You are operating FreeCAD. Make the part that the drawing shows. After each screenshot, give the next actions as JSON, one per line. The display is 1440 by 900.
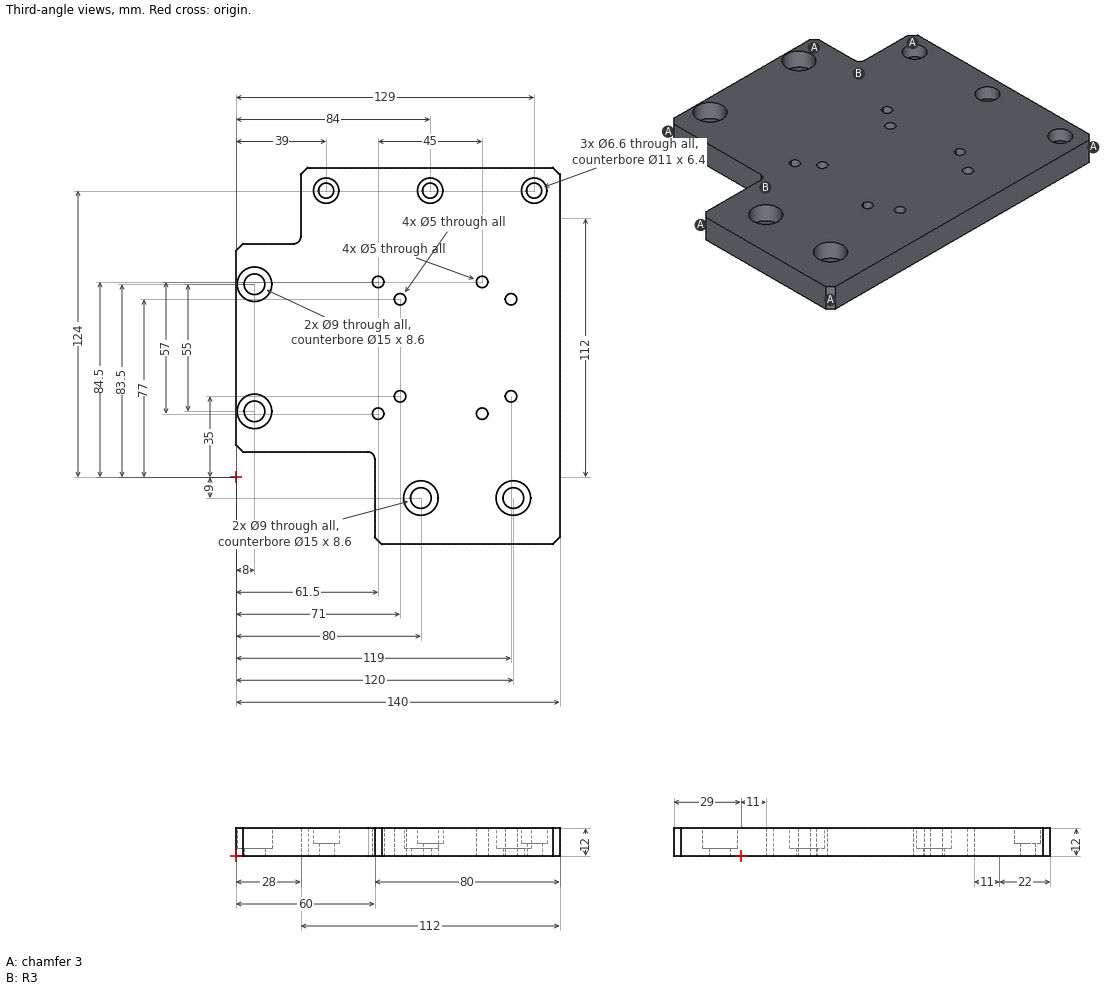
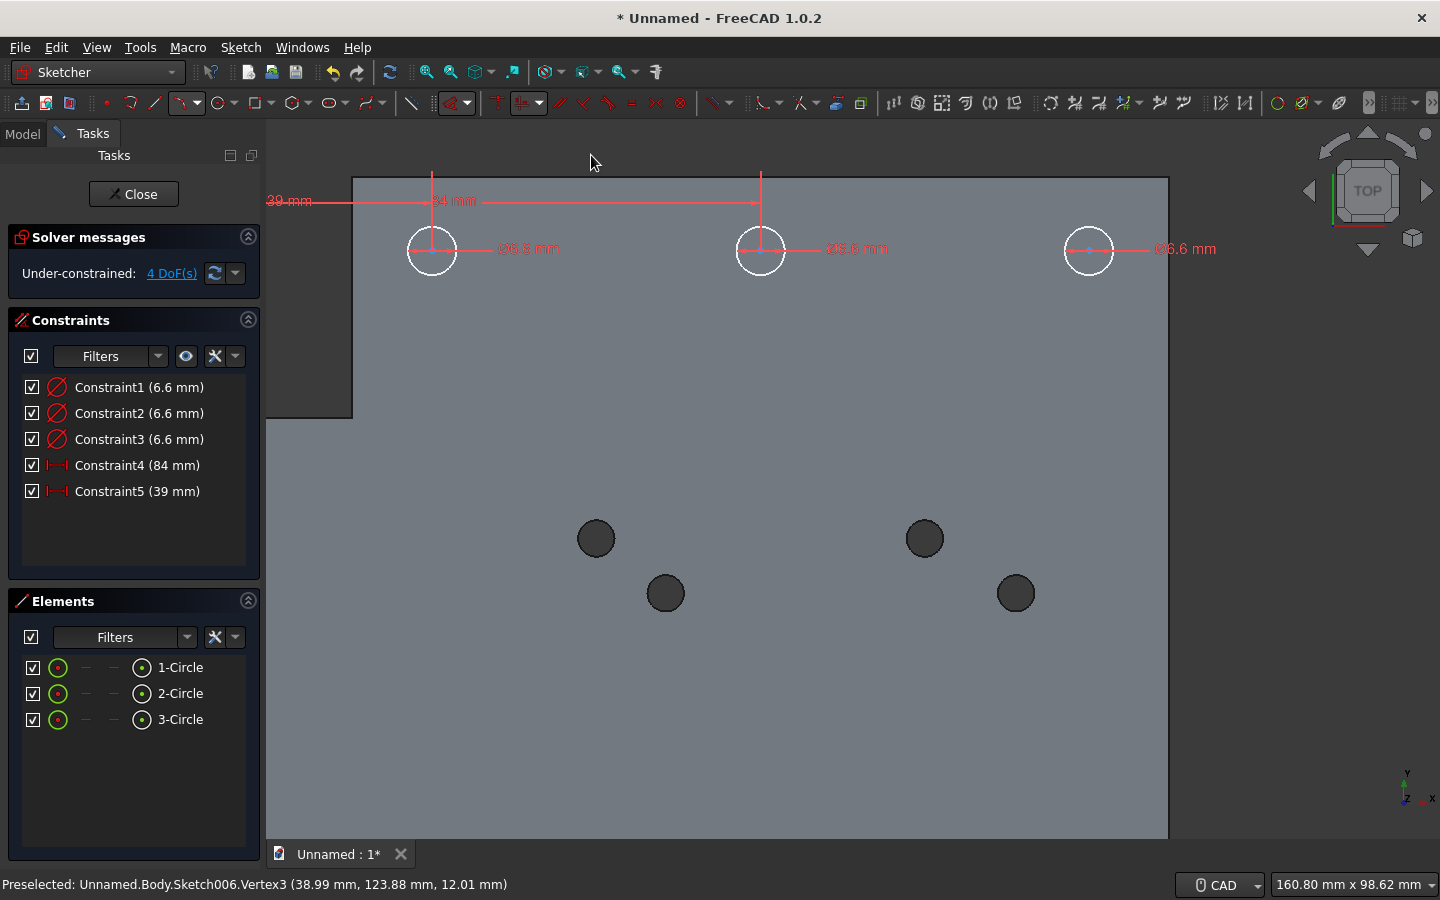
{"action": "left_click", "coordinate": [1089, 251]}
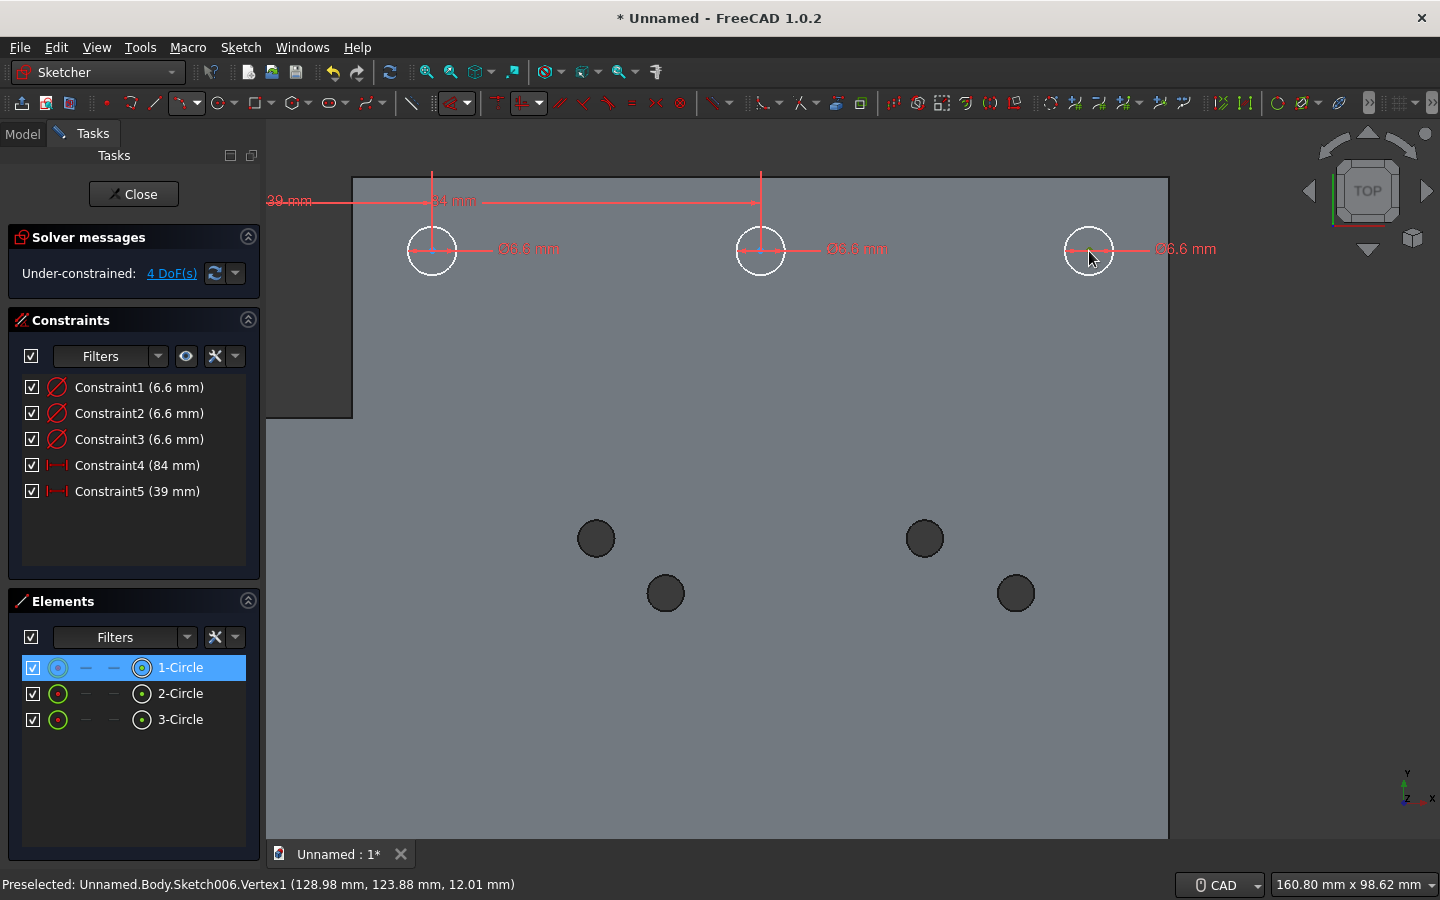
{"action": "left_click", "coordinate": [470, 104]}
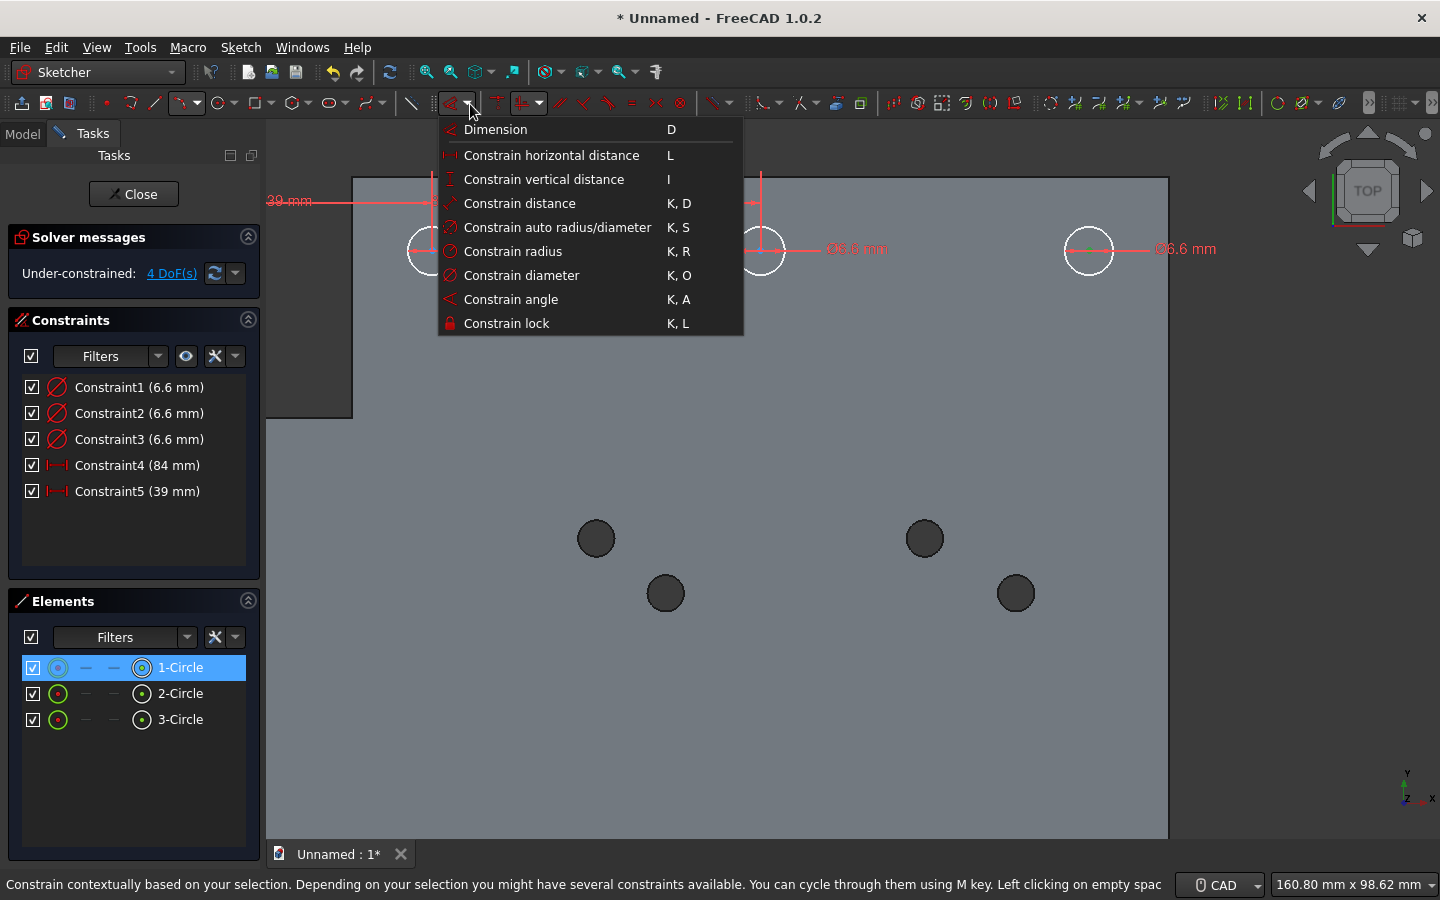
{"action": "left_click", "coordinate": [591, 155]}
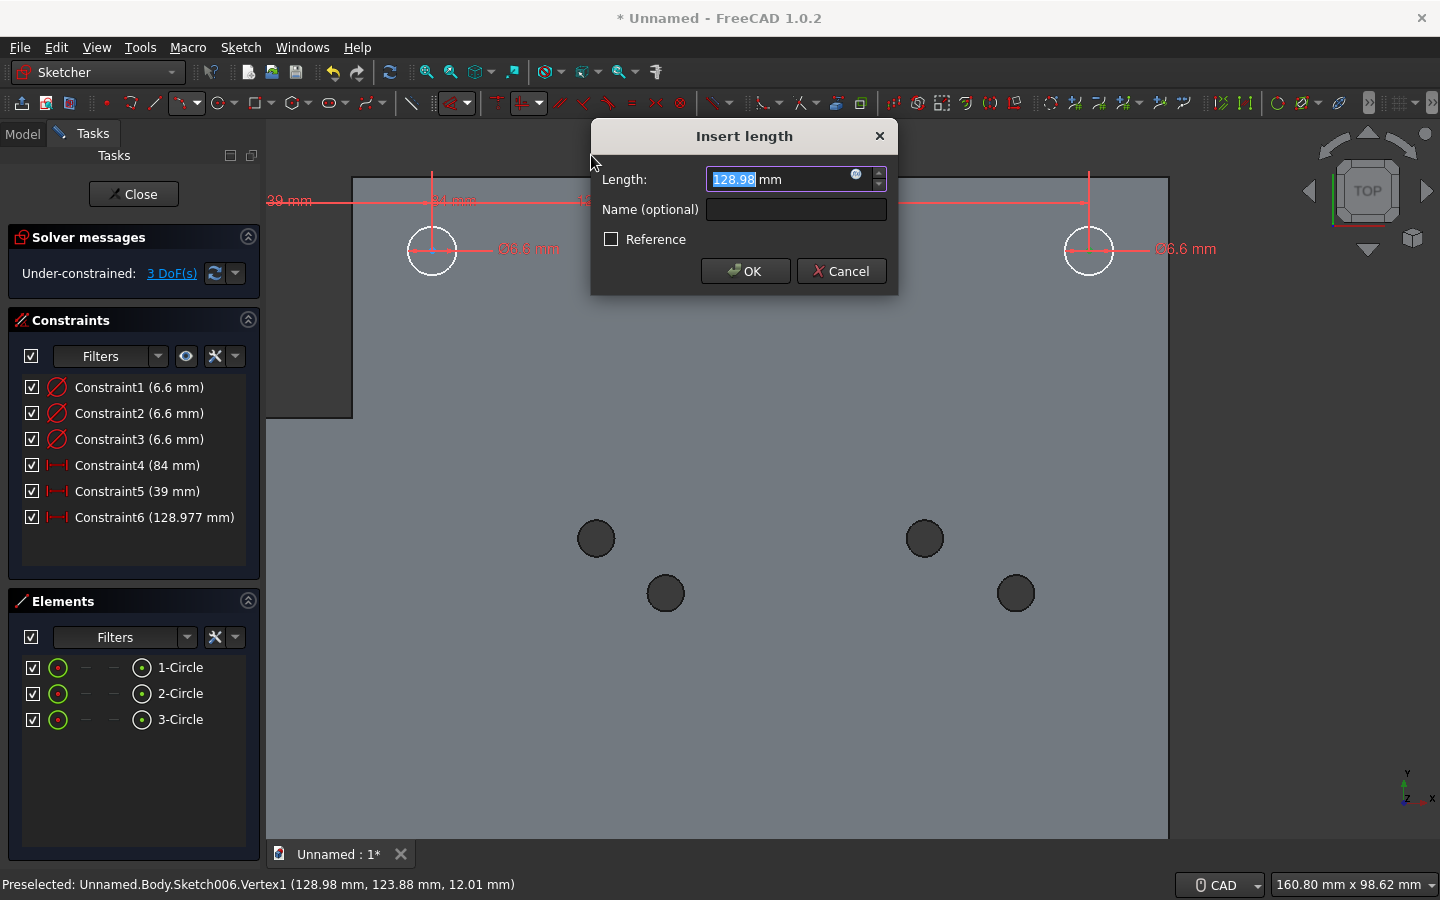
{"action": "type", "text": "129"}
{"action": "key", "text": "Return"}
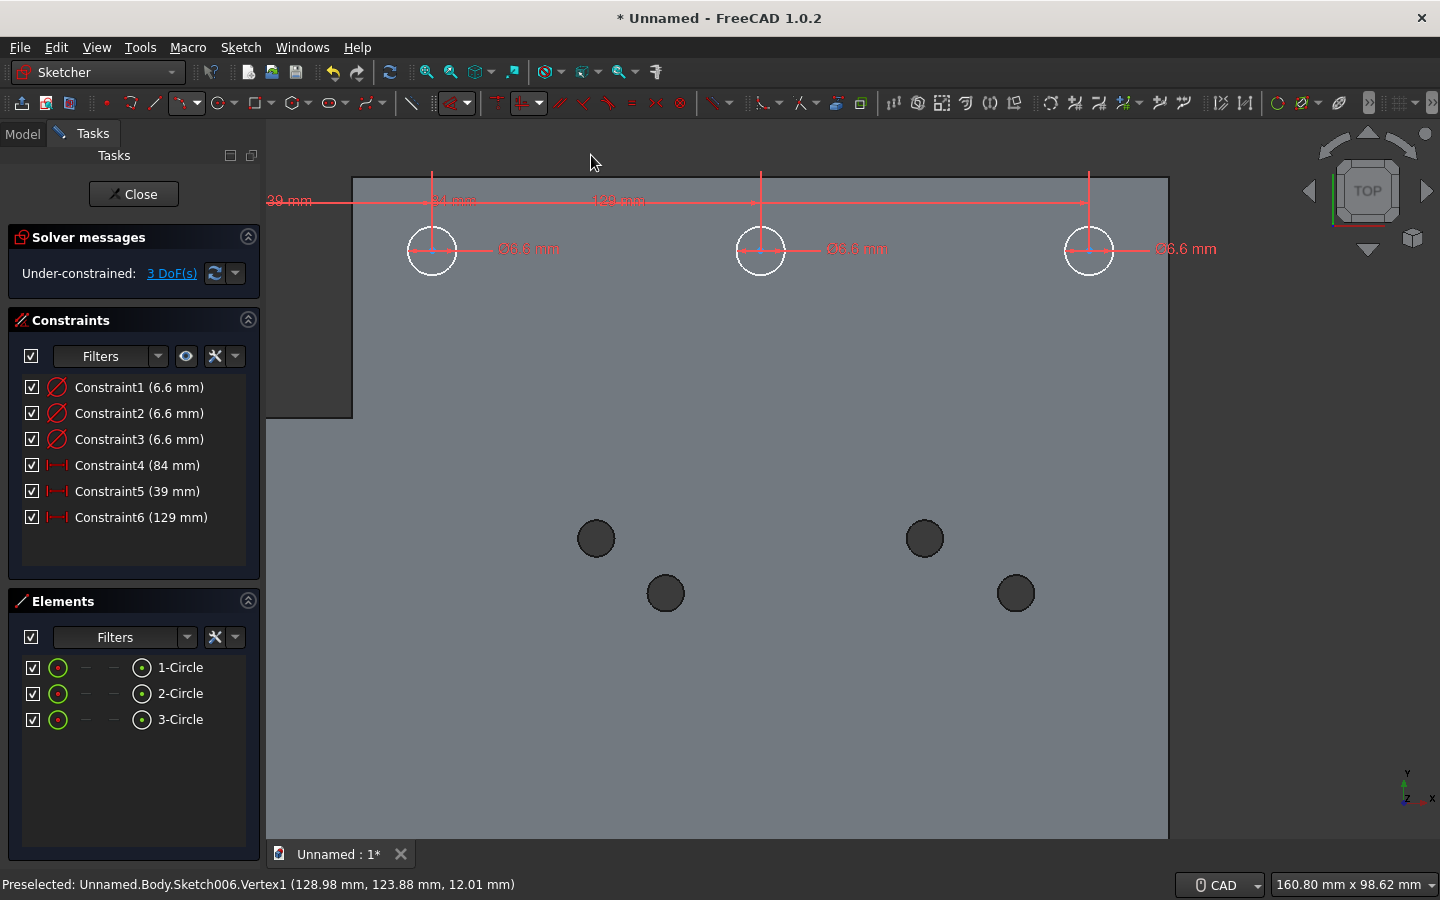
{"action": "left_click", "coordinate": [1089, 251]}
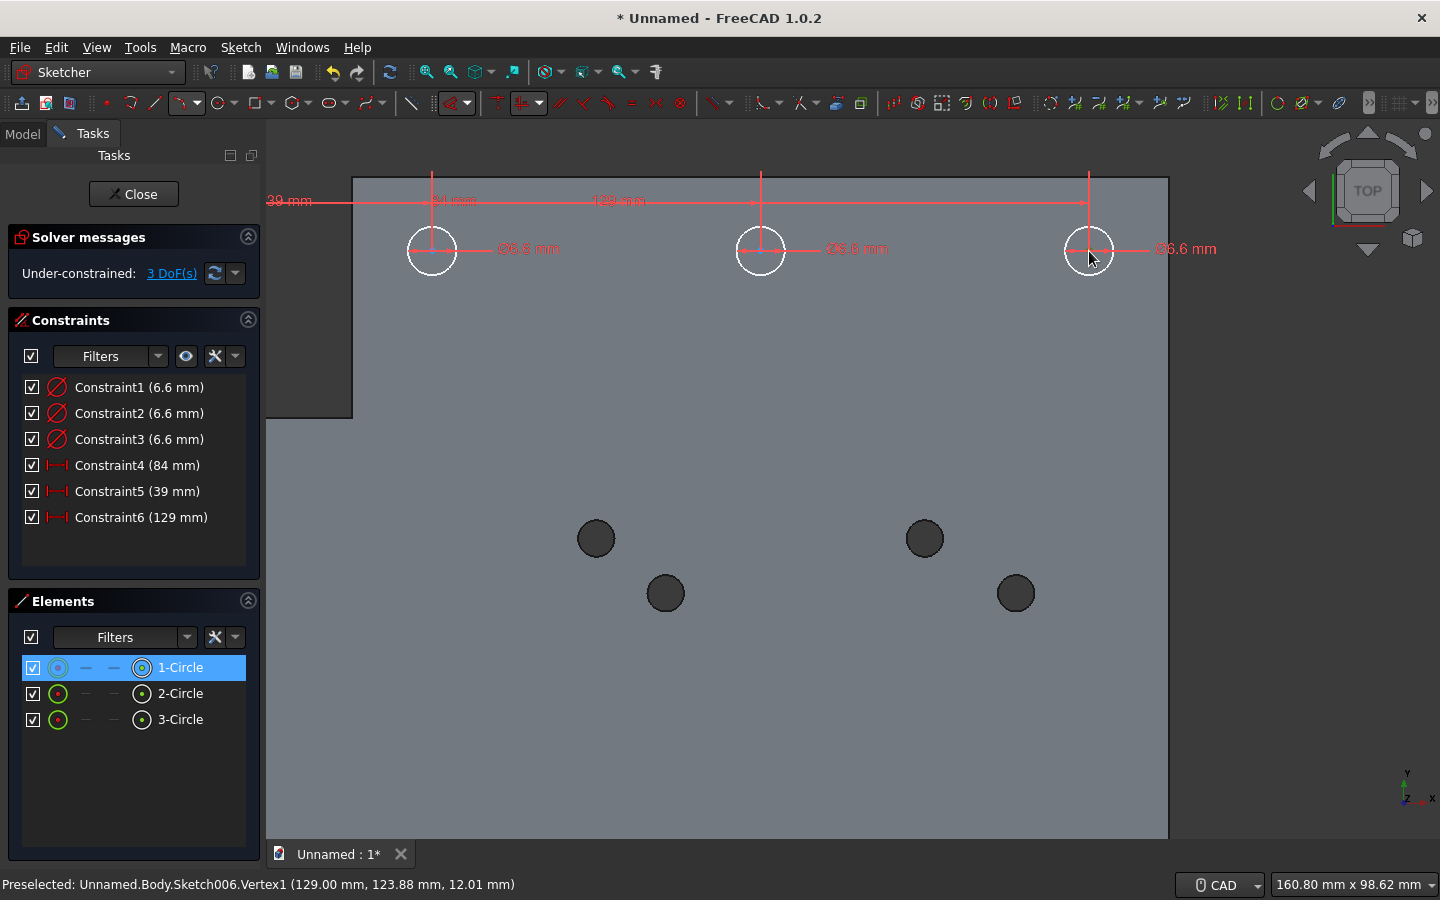
{"action": "left_click", "coordinate": [470, 104]}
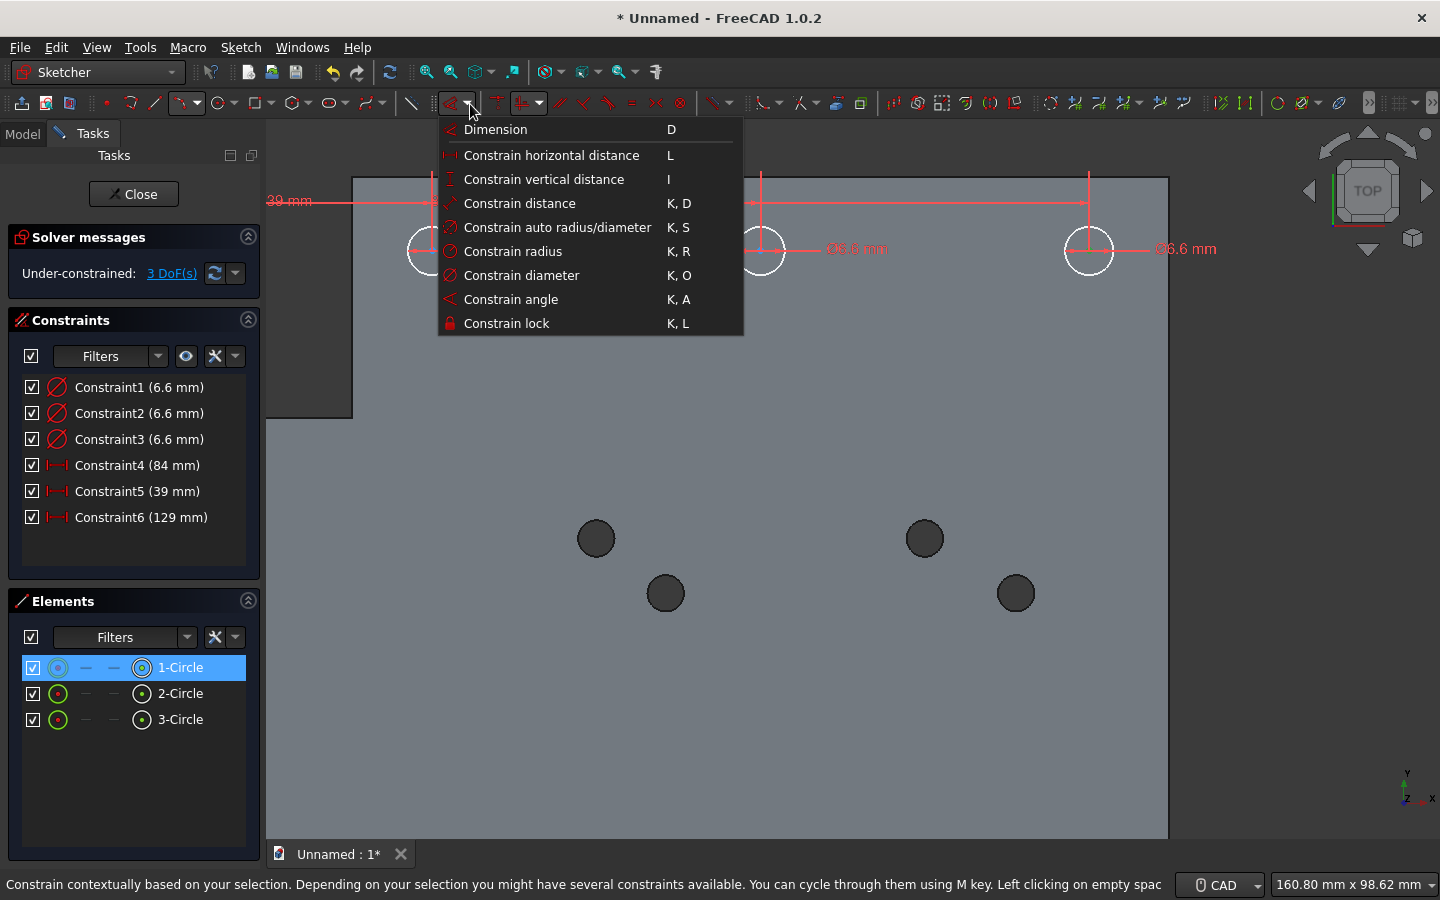
{"action": "left_click", "coordinate": [591, 179]}